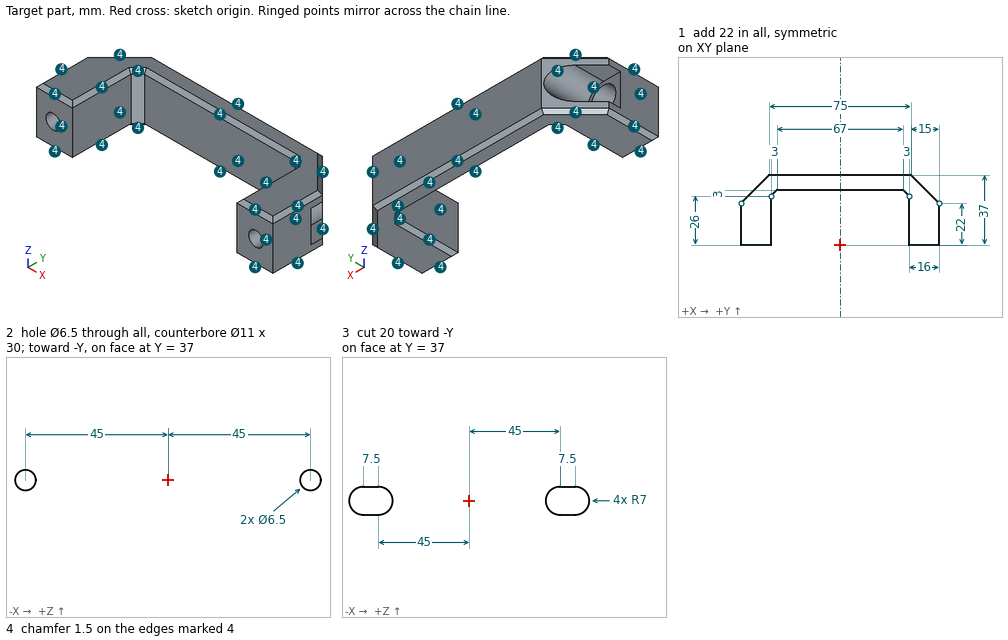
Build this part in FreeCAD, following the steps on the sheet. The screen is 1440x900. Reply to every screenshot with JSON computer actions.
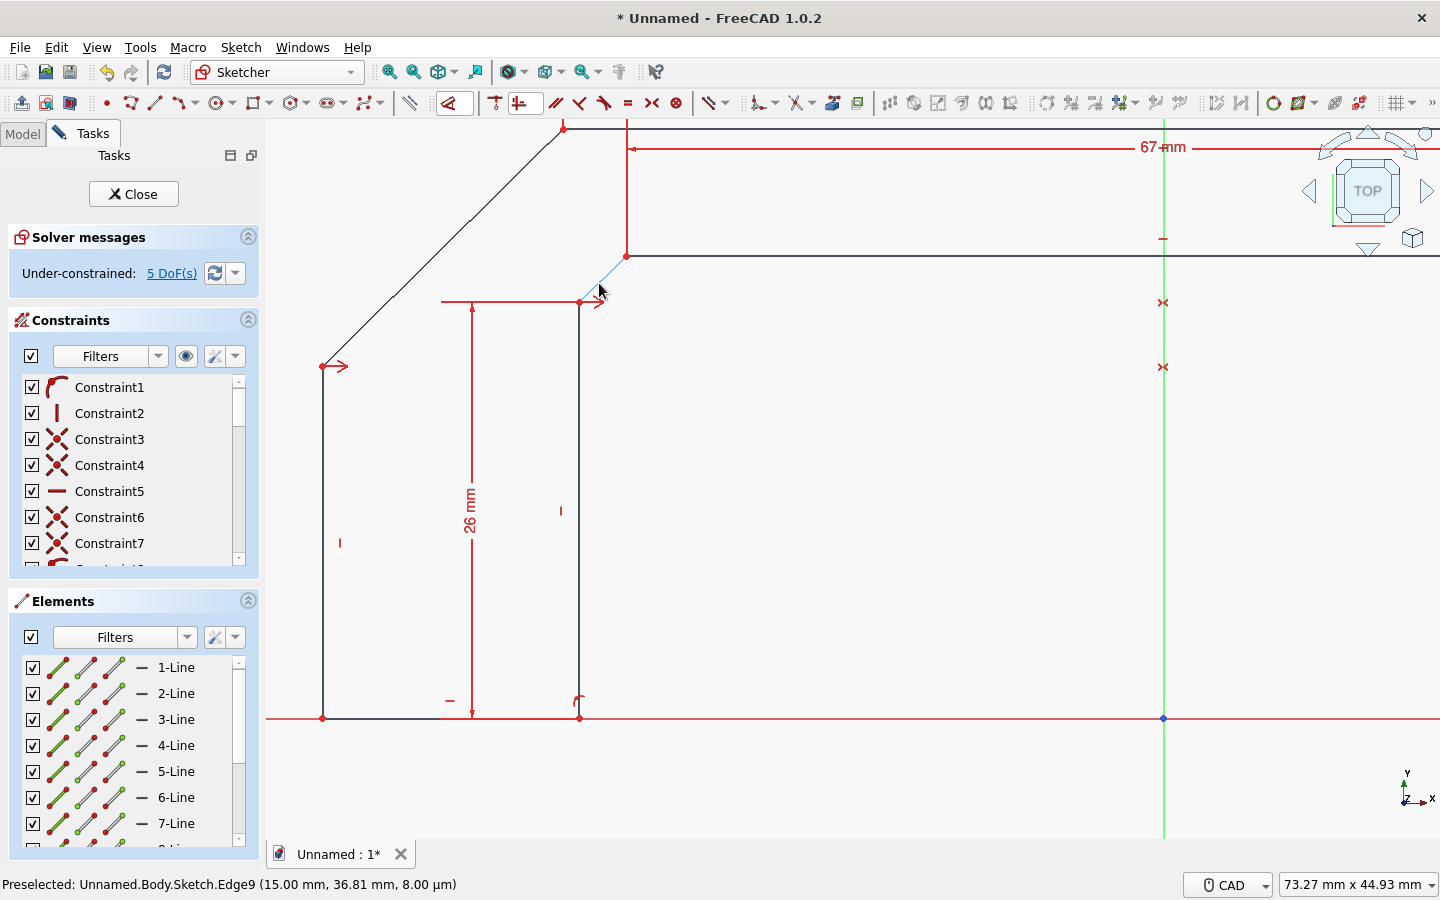
{"action": "left_click", "coordinate": [598, 284]}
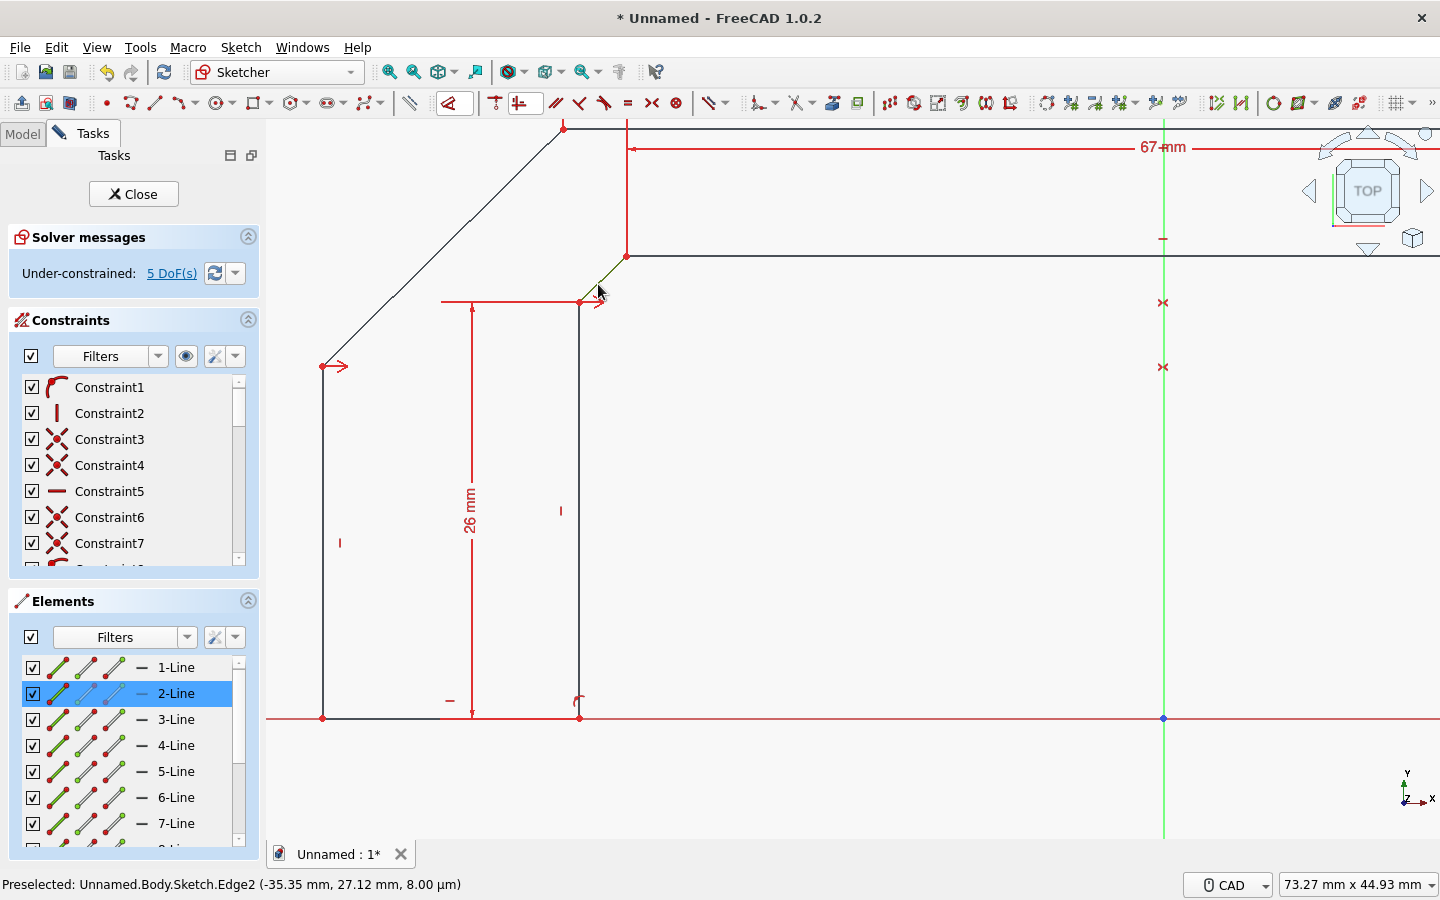
{"action": "left_click", "coordinate": [468, 104]}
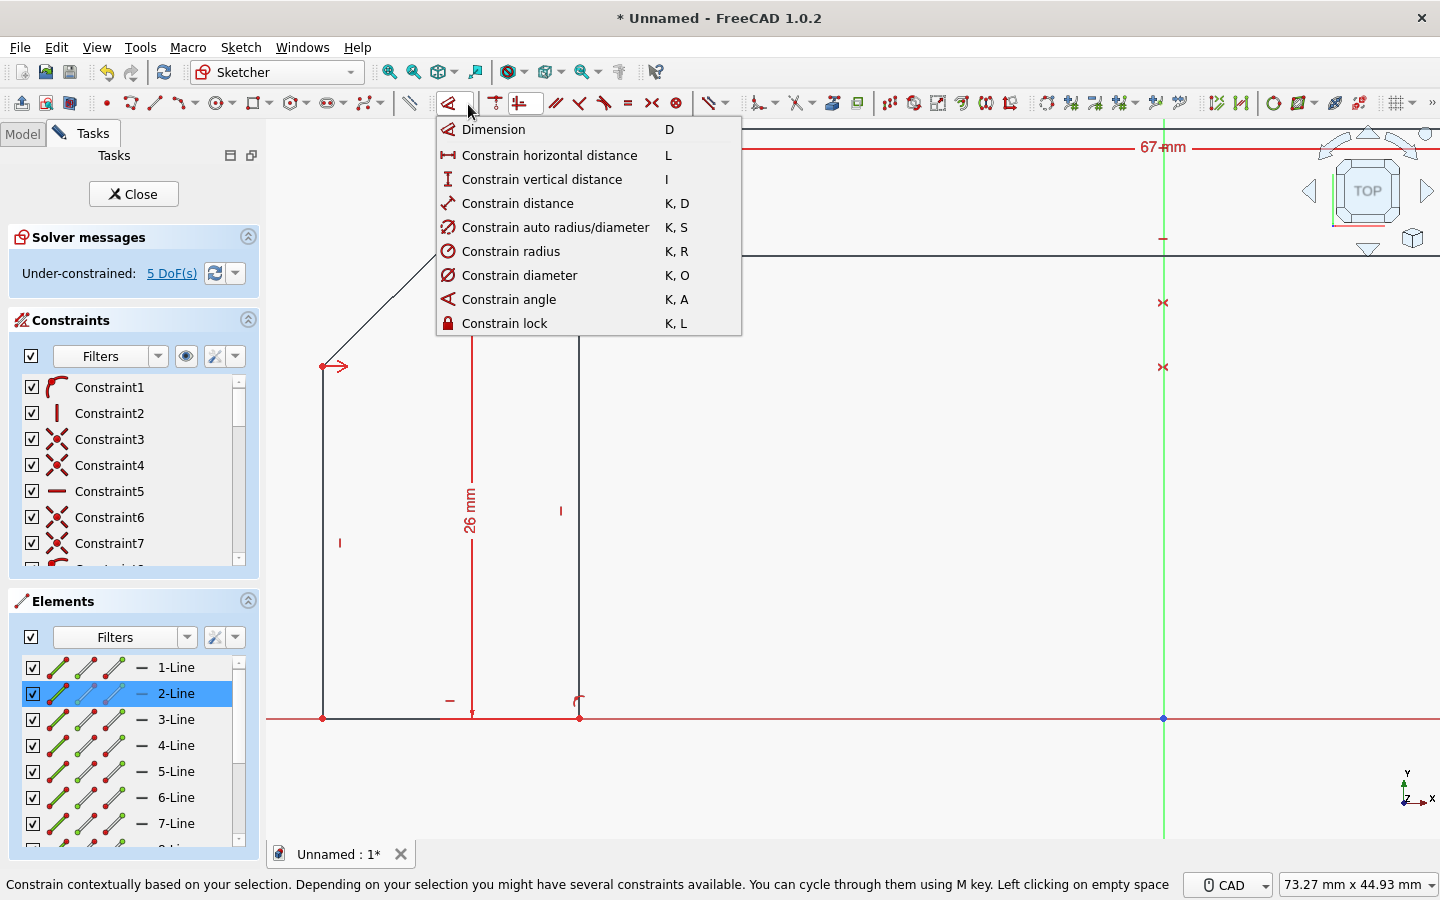
{"action": "left_click", "coordinate": [589, 155]}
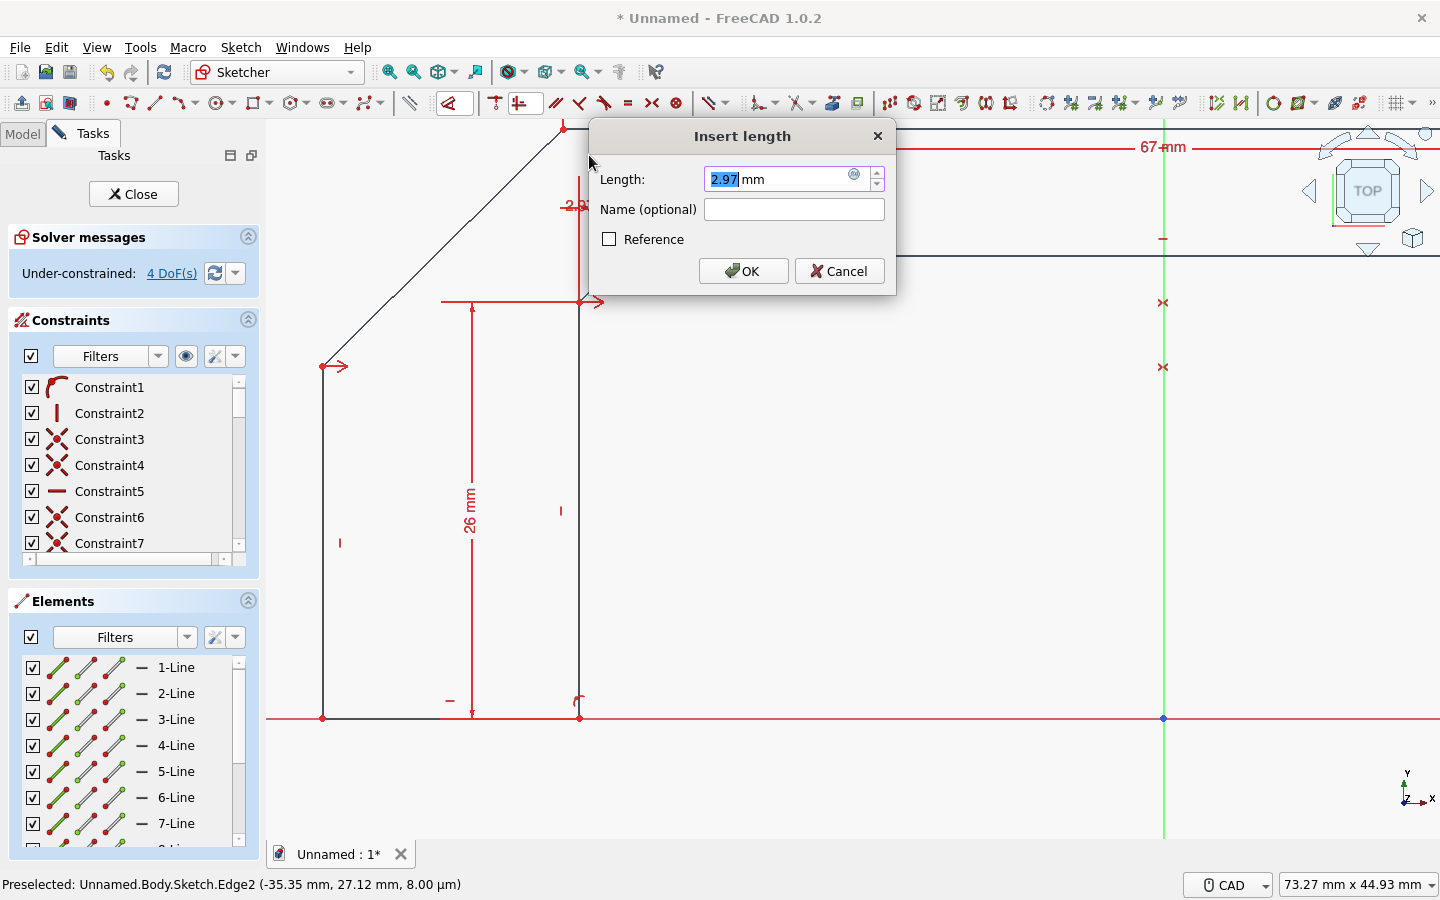
{"action": "type", "text": "3"}
{"action": "key", "text": "Return"}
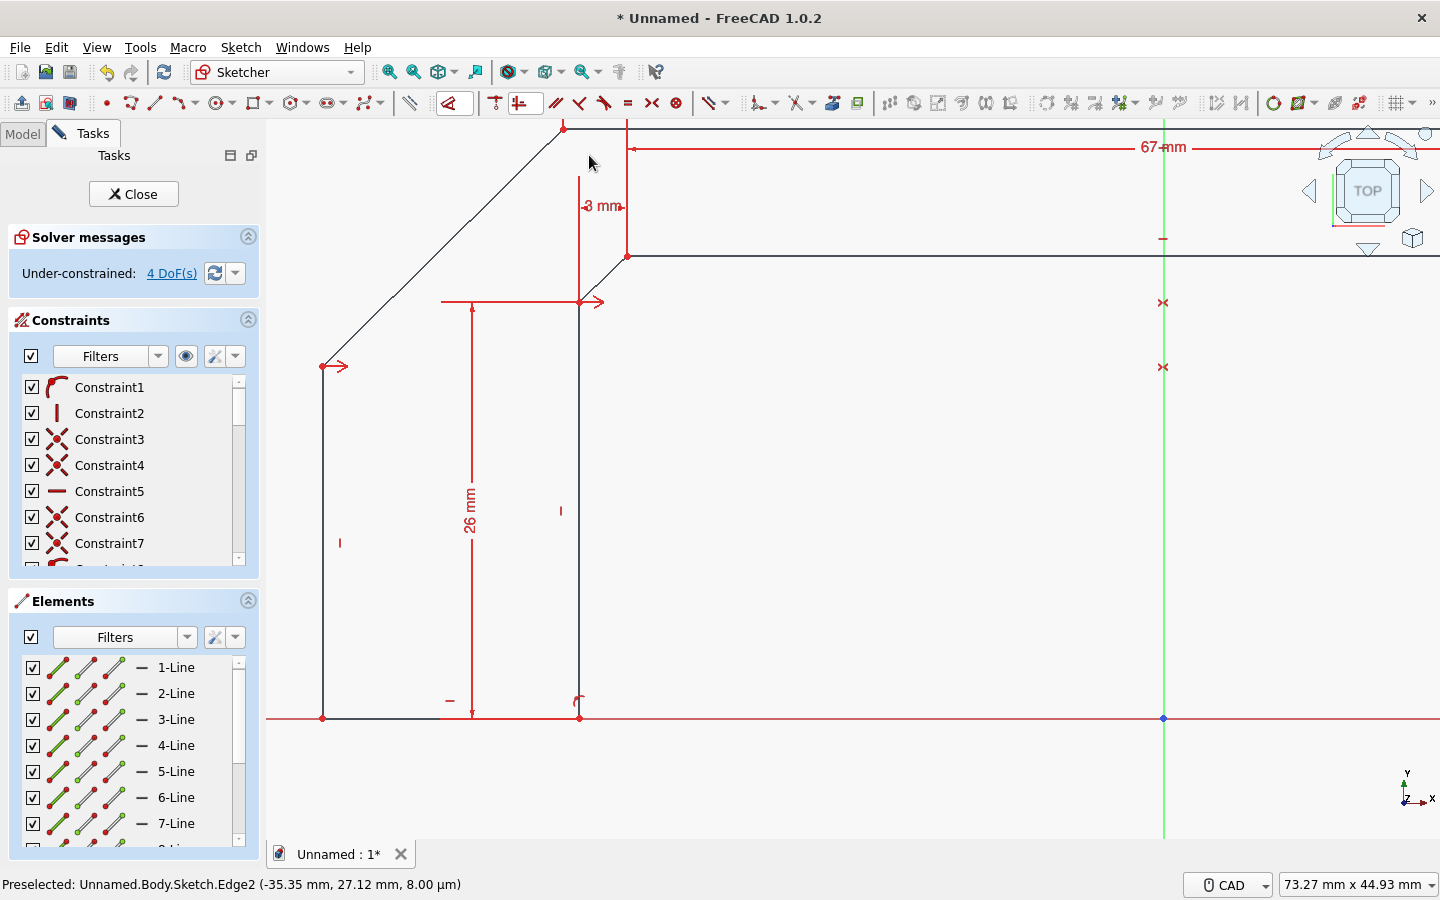
{"action": "left_click", "coordinate": [593, 288]}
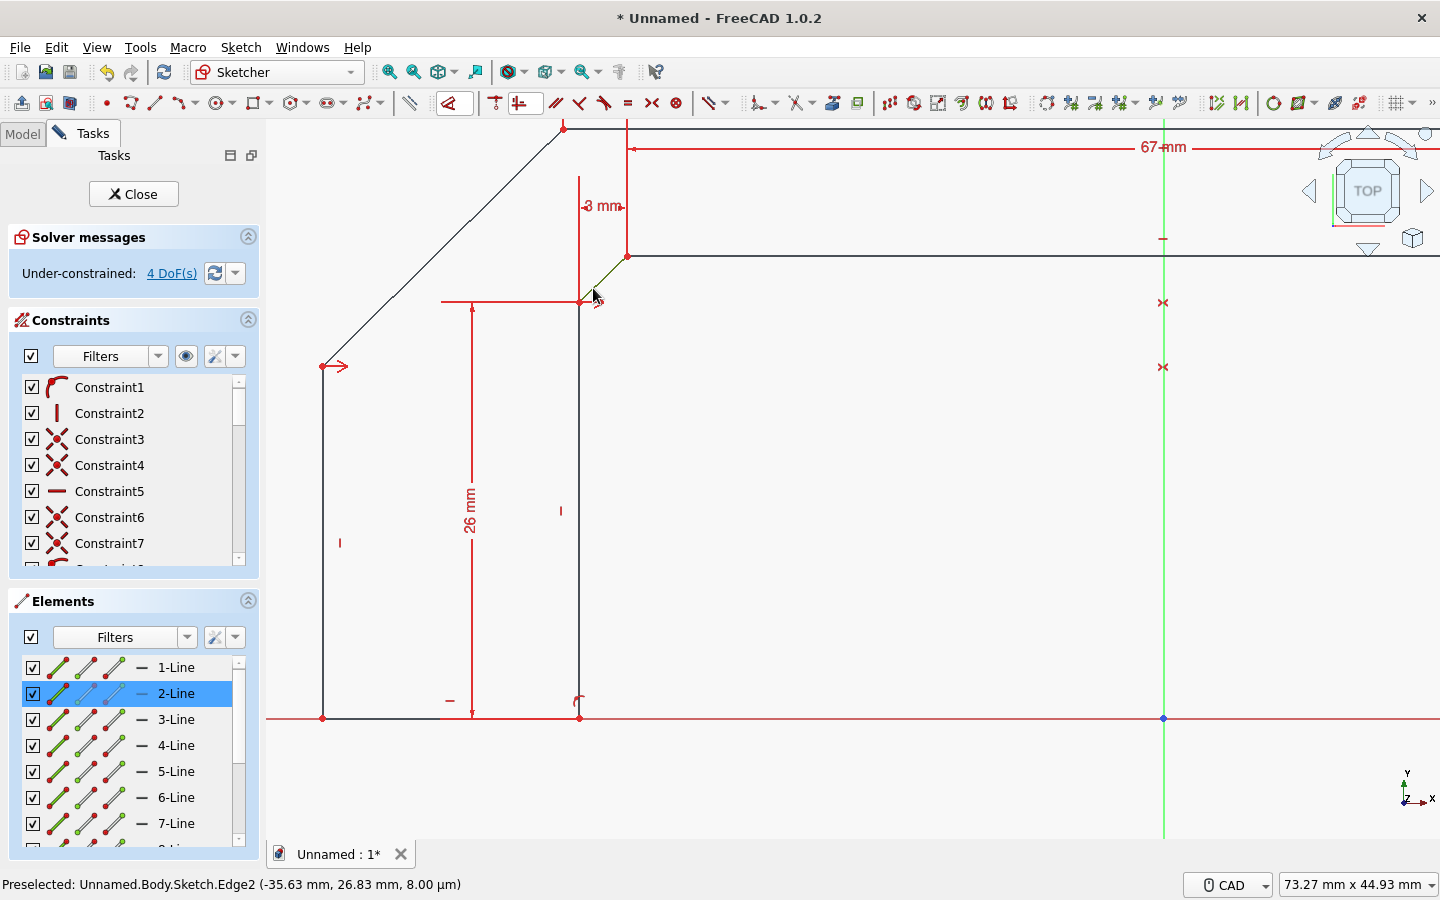
{"action": "key", "text": "i"}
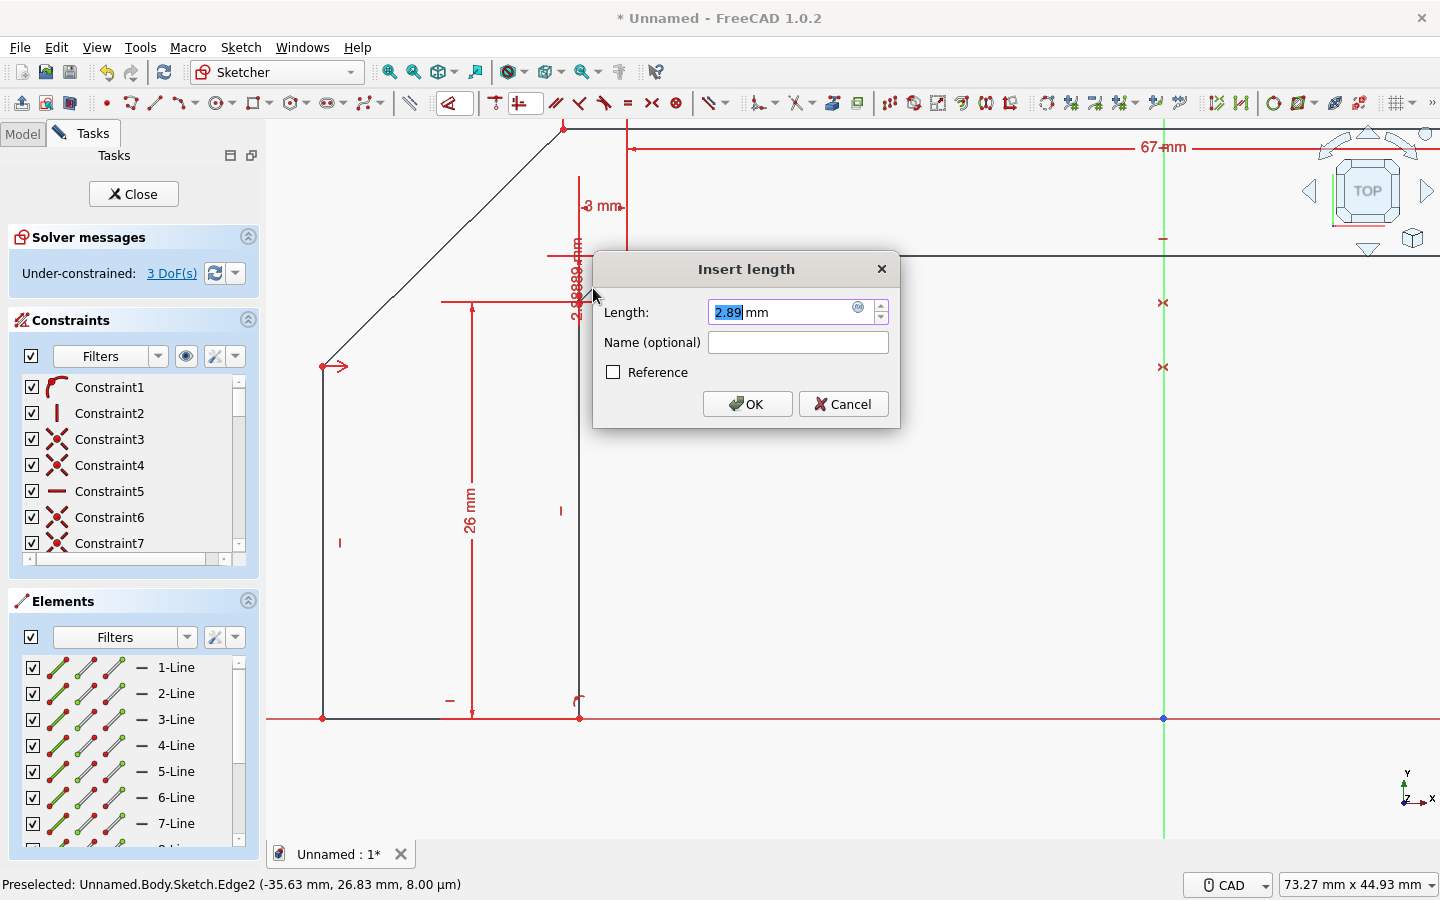
{"action": "type", "text": "3"}
{"action": "key", "text": "Return"}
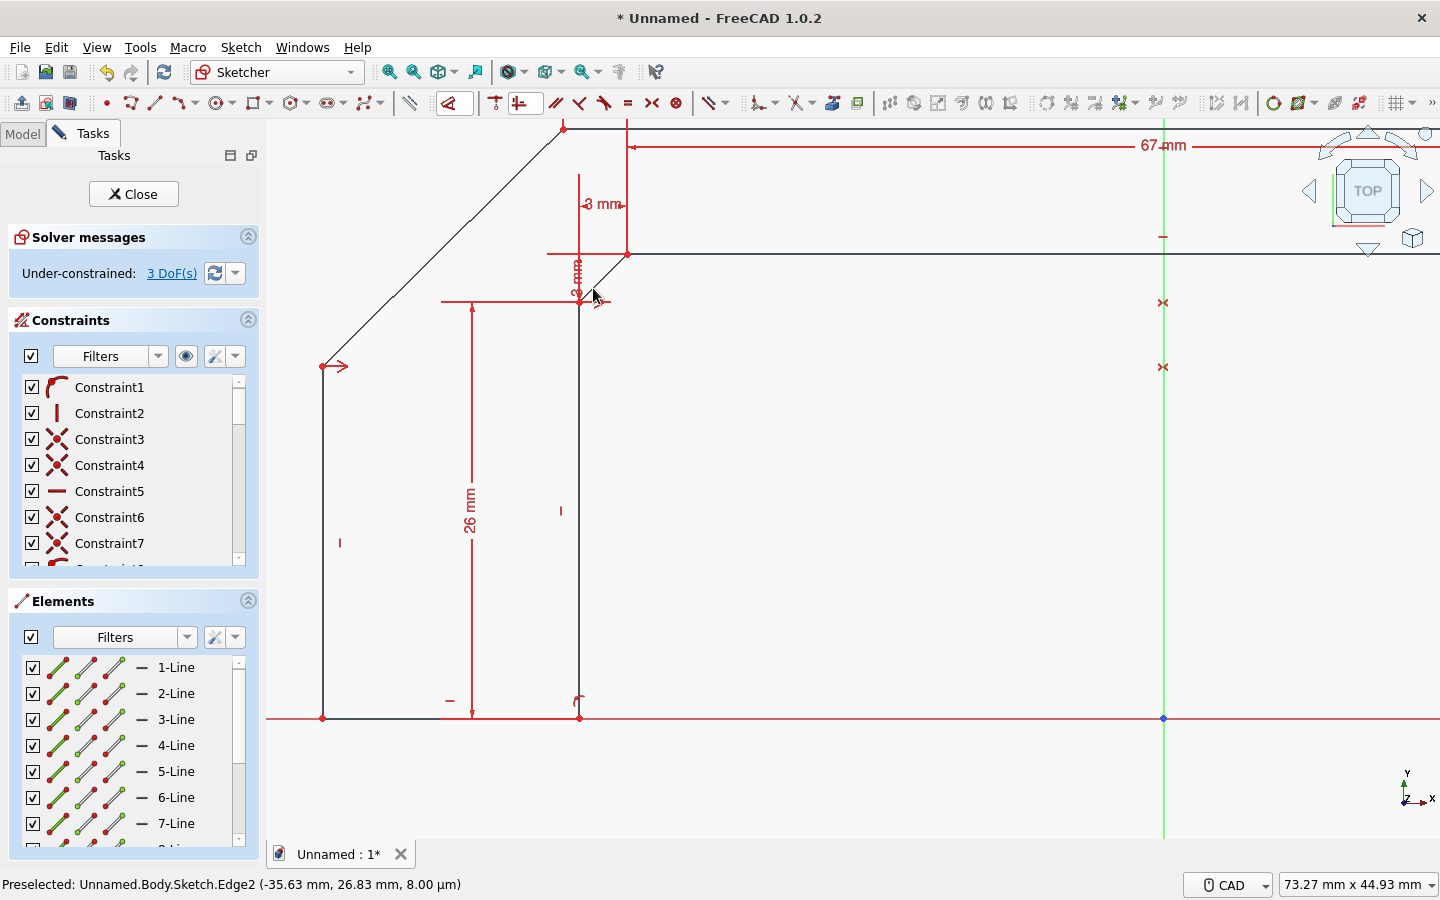
{"action": "scroll", "coordinate": [475, 525], "scroll_direction": "down", "scroll_amount": 4}